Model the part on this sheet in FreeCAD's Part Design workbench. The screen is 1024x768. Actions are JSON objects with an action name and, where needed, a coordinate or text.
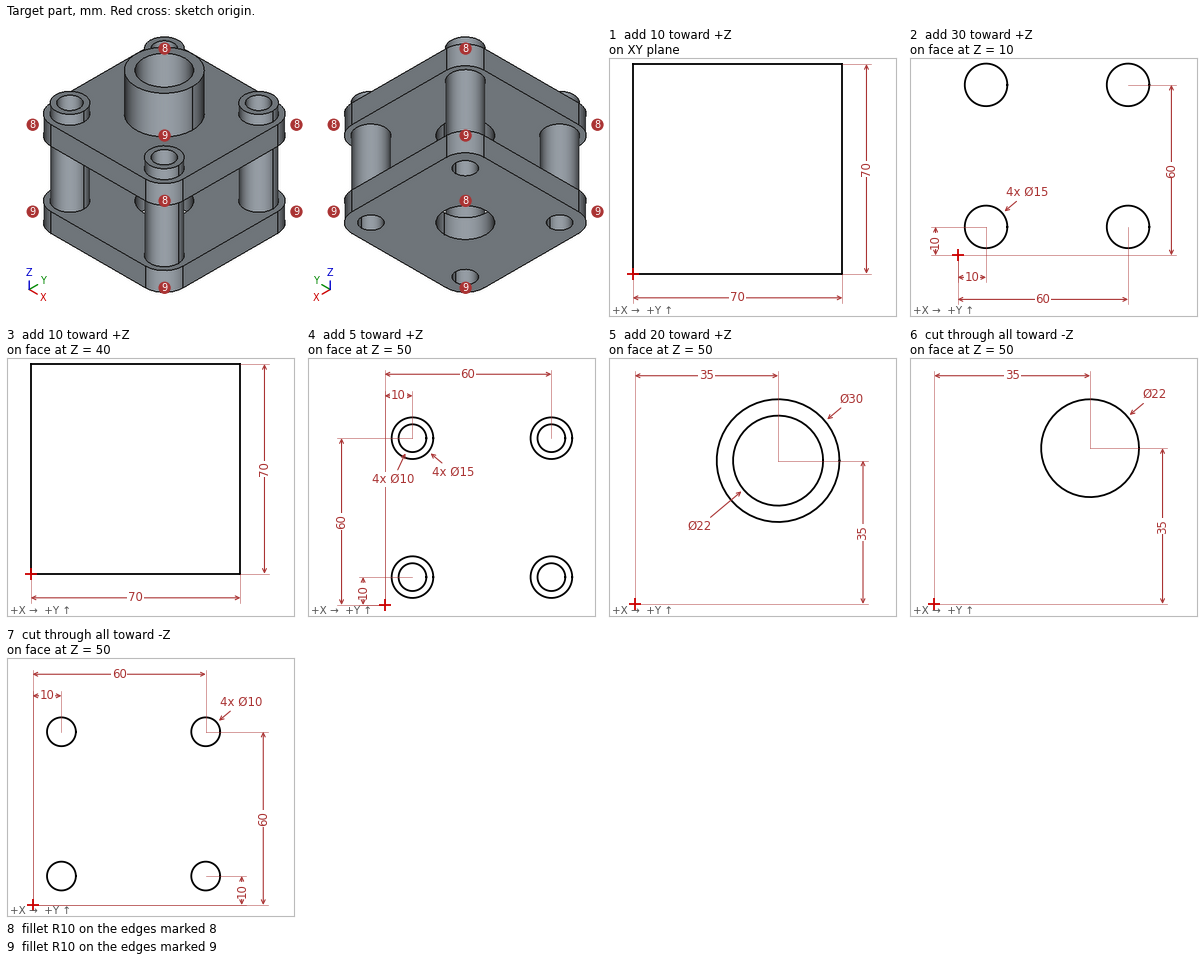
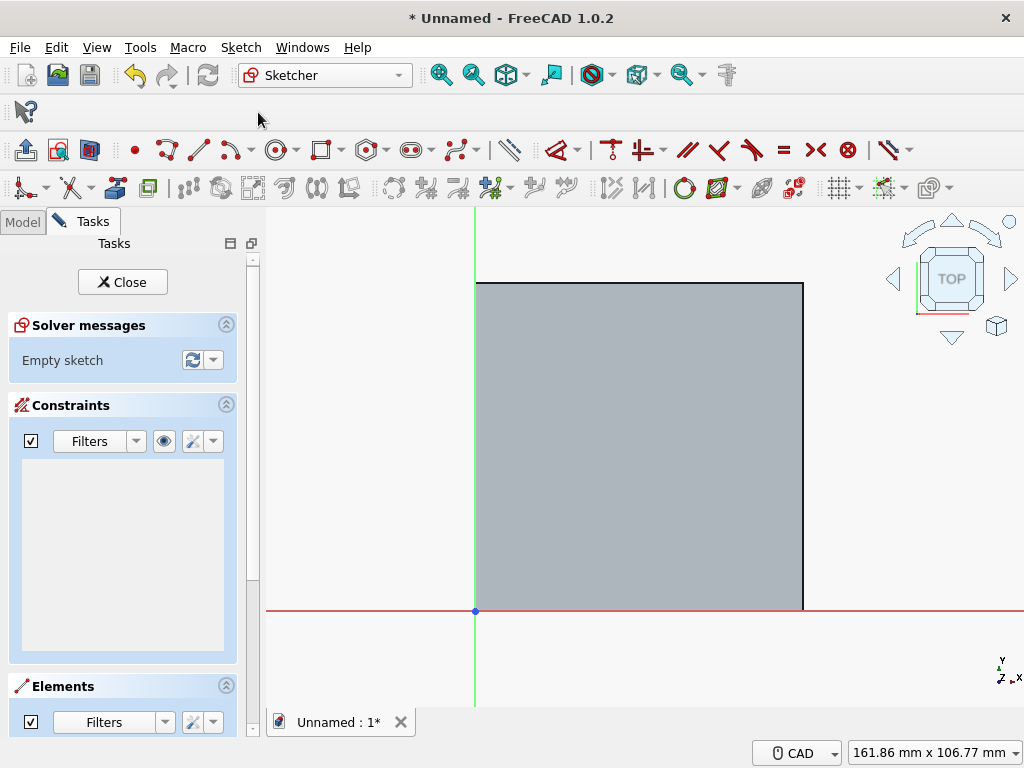
{"action": "left_click", "coordinate": [276, 150]}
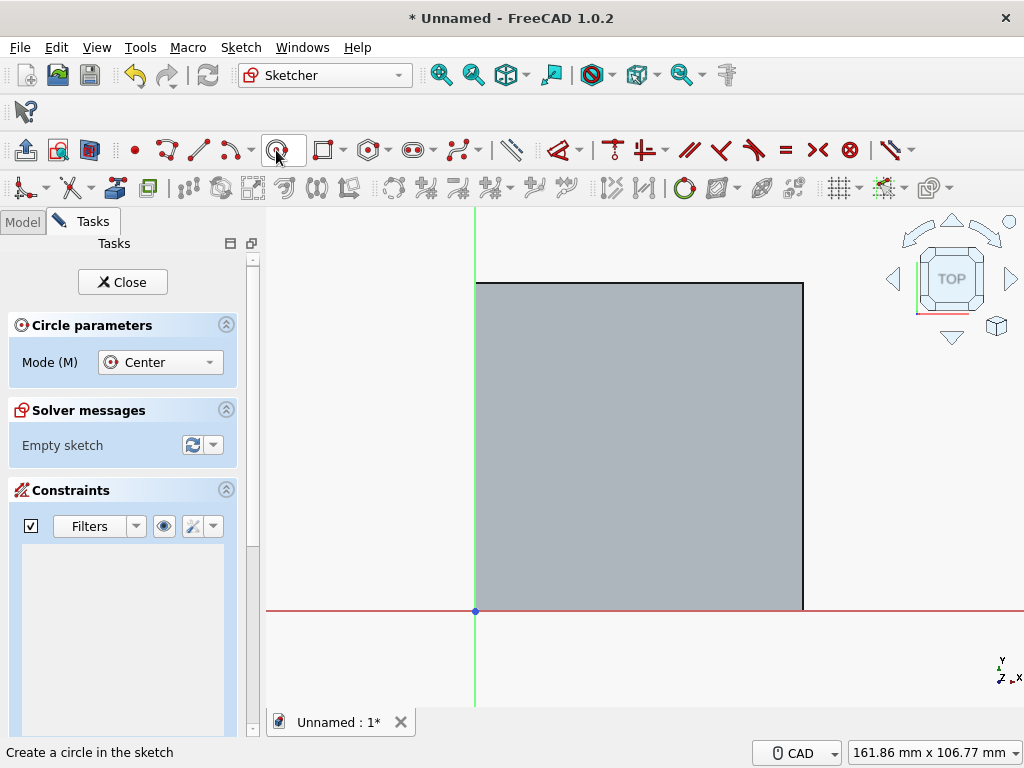
{"action": "left_click", "coordinate": [522, 330]}
{"action": "left_click", "coordinate": [547, 305]}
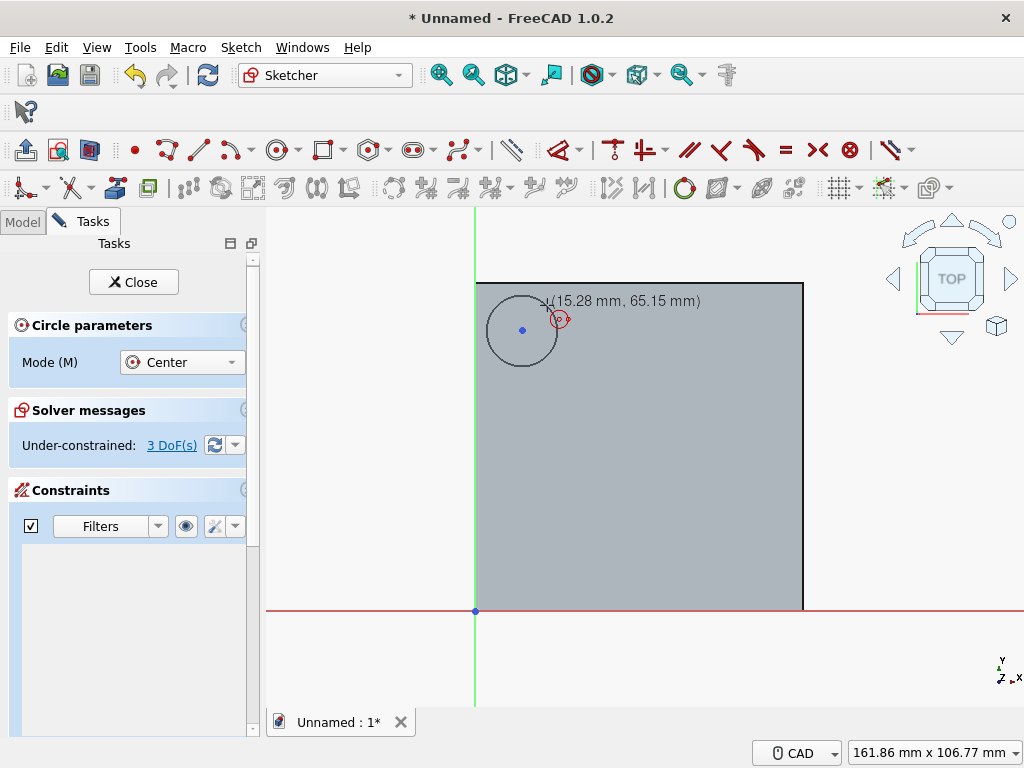
{"action": "left_click", "coordinate": [756, 330]}
{"action": "left_click", "coordinate": [781, 305]}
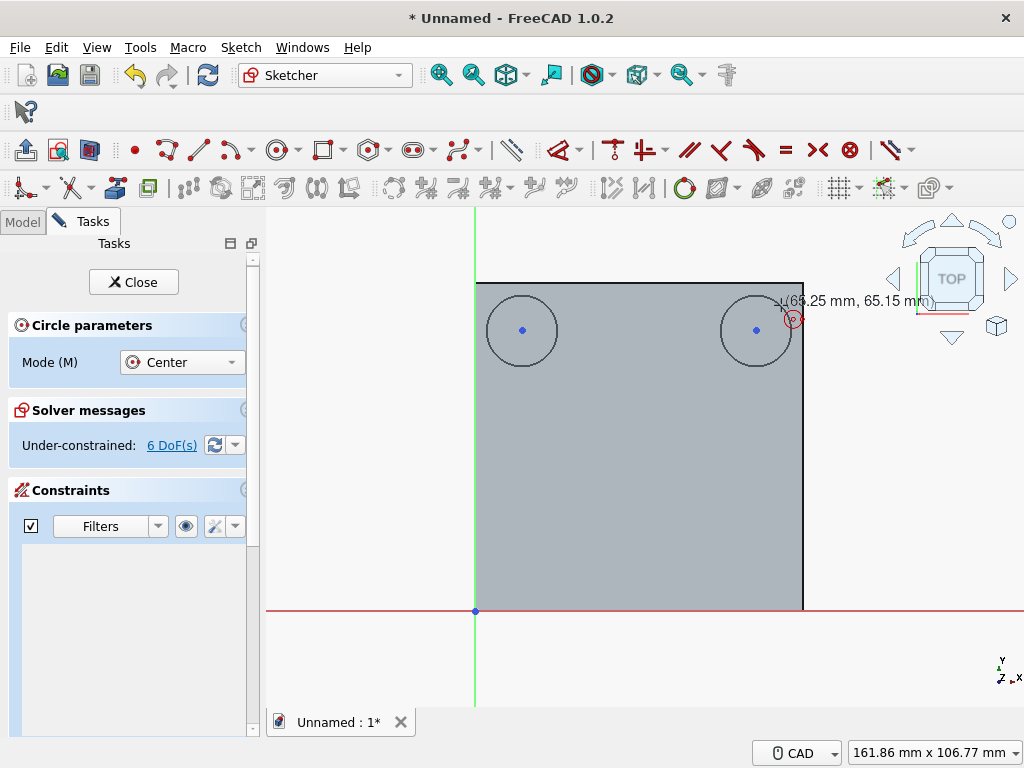
{"action": "left_click", "coordinate": [522, 564]}
{"action": "left_click", "coordinate": [547, 539]}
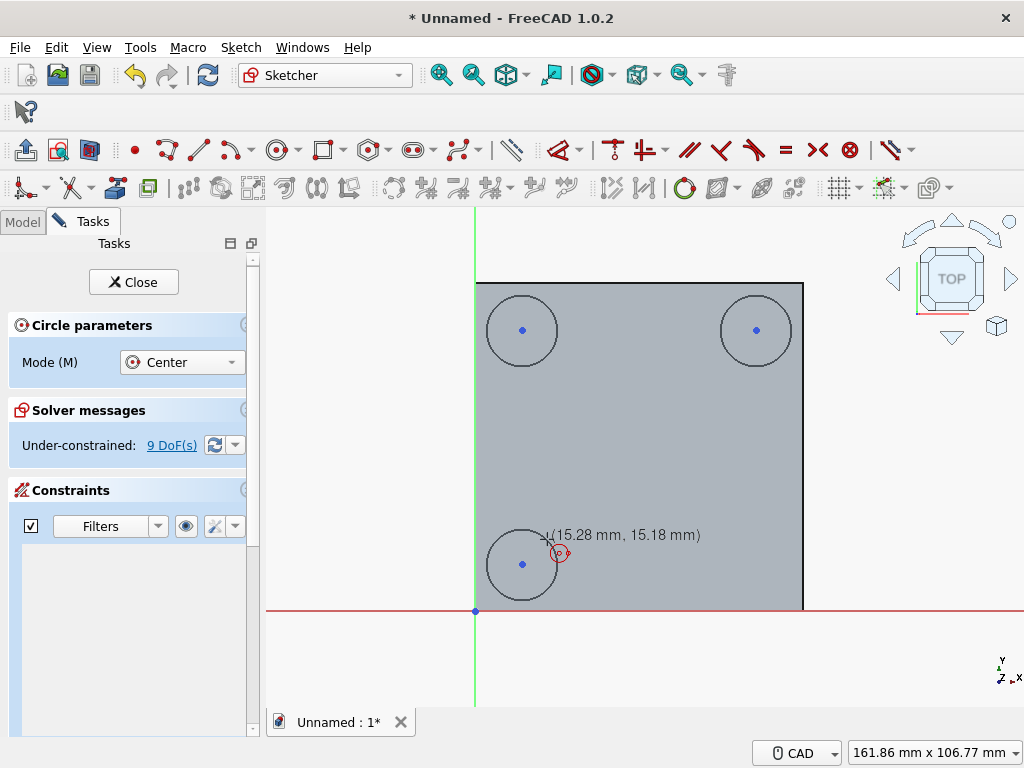
{"action": "left_click", "coordinate": [756, 564]}
{"action": "left_click", "coordinate": [781, 539]}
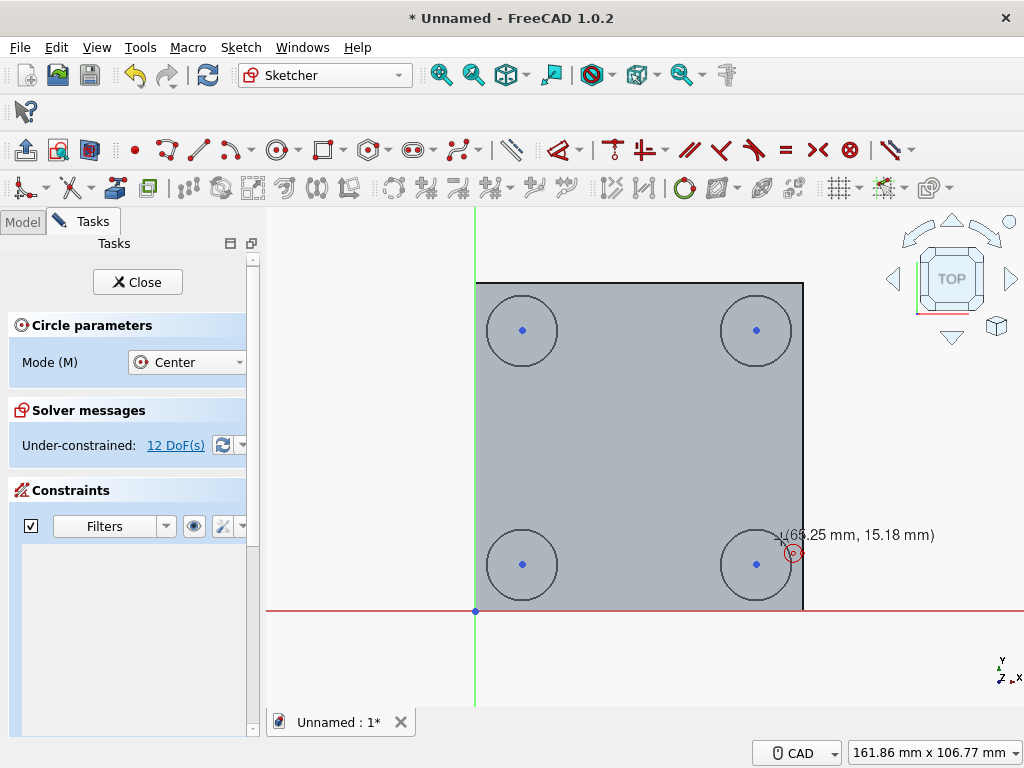
{"action": "left_click", "coordinate": [522, 331]}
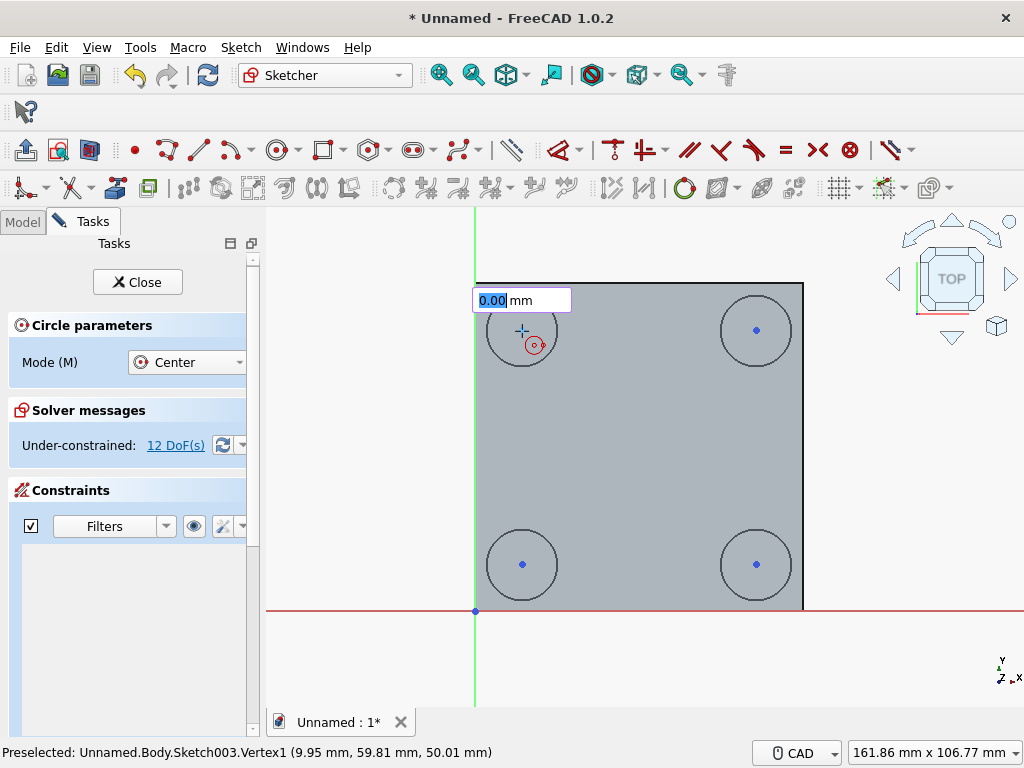
{"action": "scroll", "coordinate": [530, 308], "scroll_direction": "up", "scroll_amount": 2}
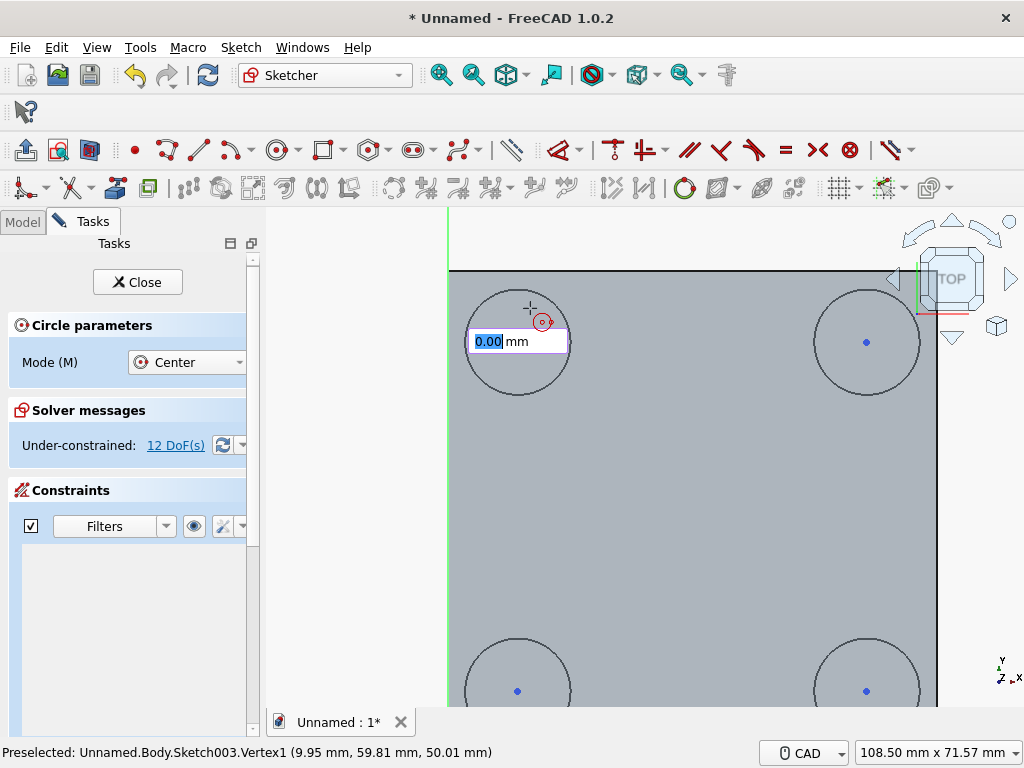
{"action": "left_click", "coordinate": [530, 308]}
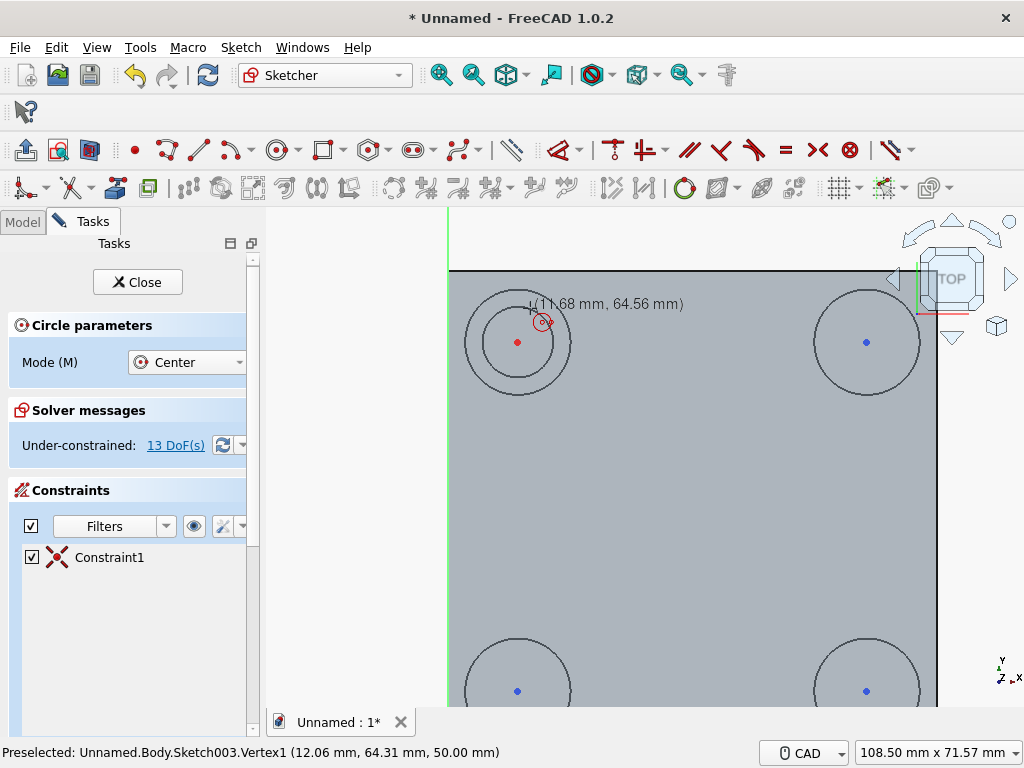
{"action": "scroll", "coordinate": [358, 320], "scroll_direction": "down", "scroll_amount": 2}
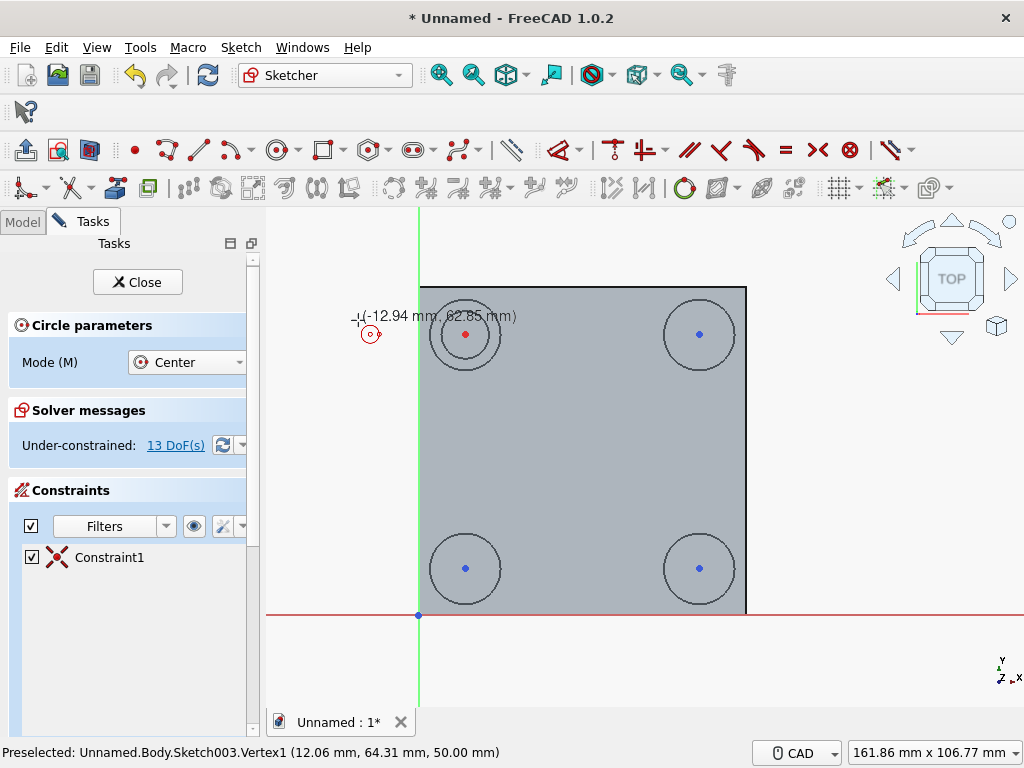
{"action": "left_click", "coordinate": [699, 335]}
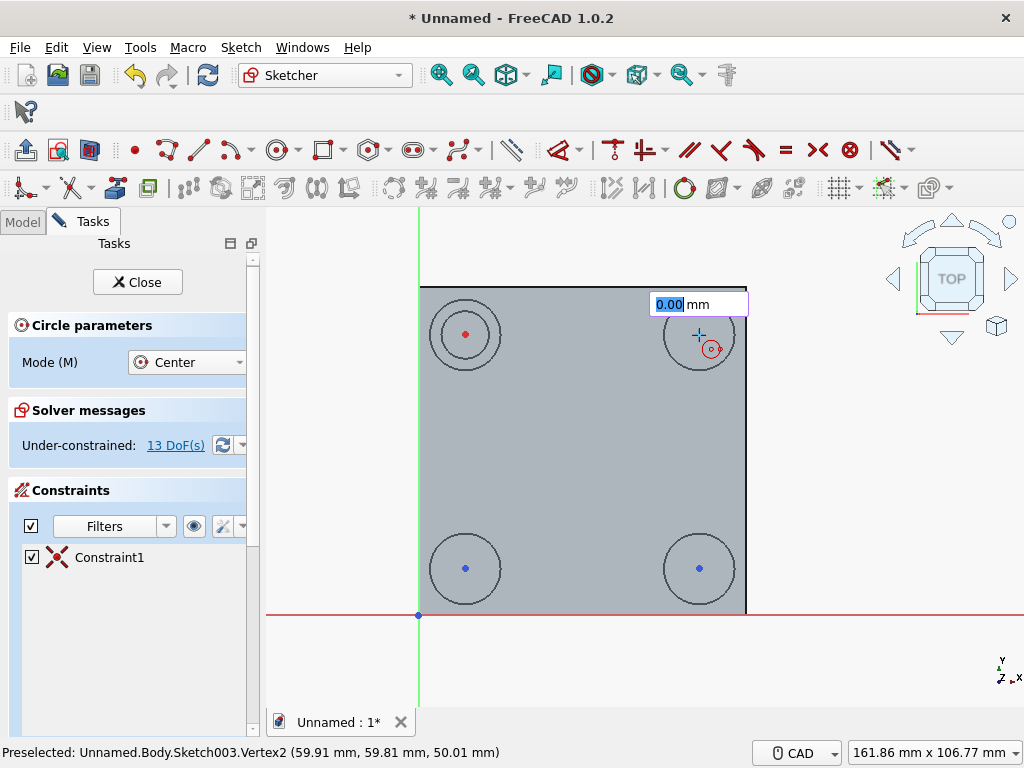
{"action": "scroll", "coordinate": [692, 356], "scroll_direction": "up", "scroll_amount": 2}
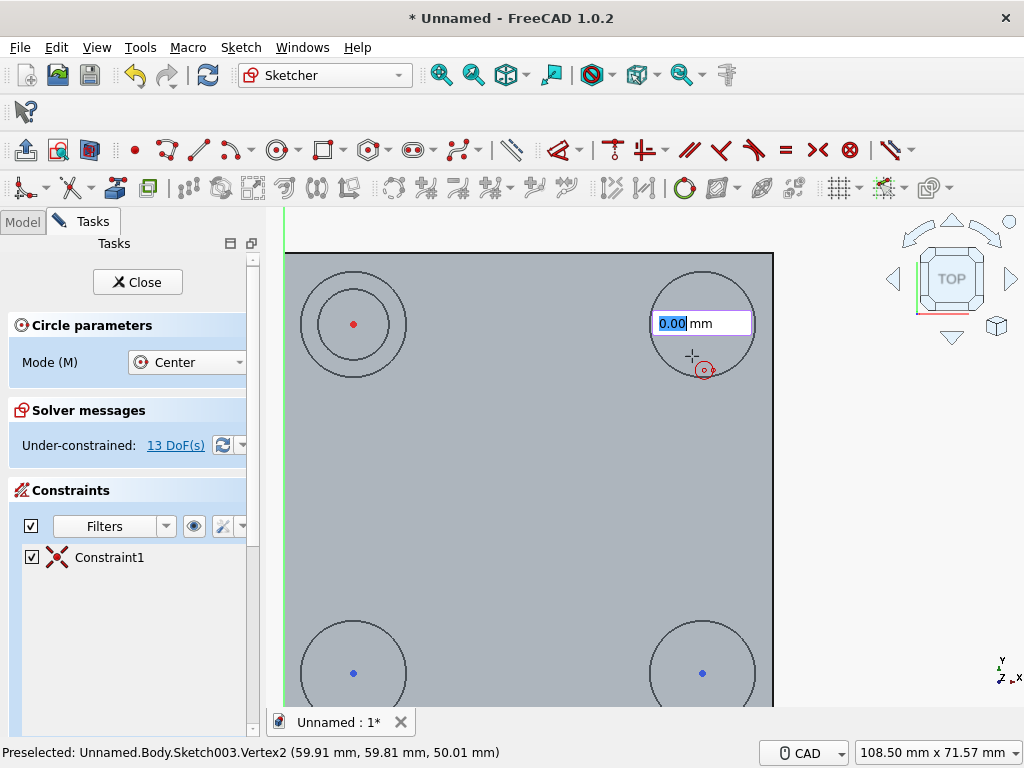
{"action": "left_click", "coordinate": [691, 356]}